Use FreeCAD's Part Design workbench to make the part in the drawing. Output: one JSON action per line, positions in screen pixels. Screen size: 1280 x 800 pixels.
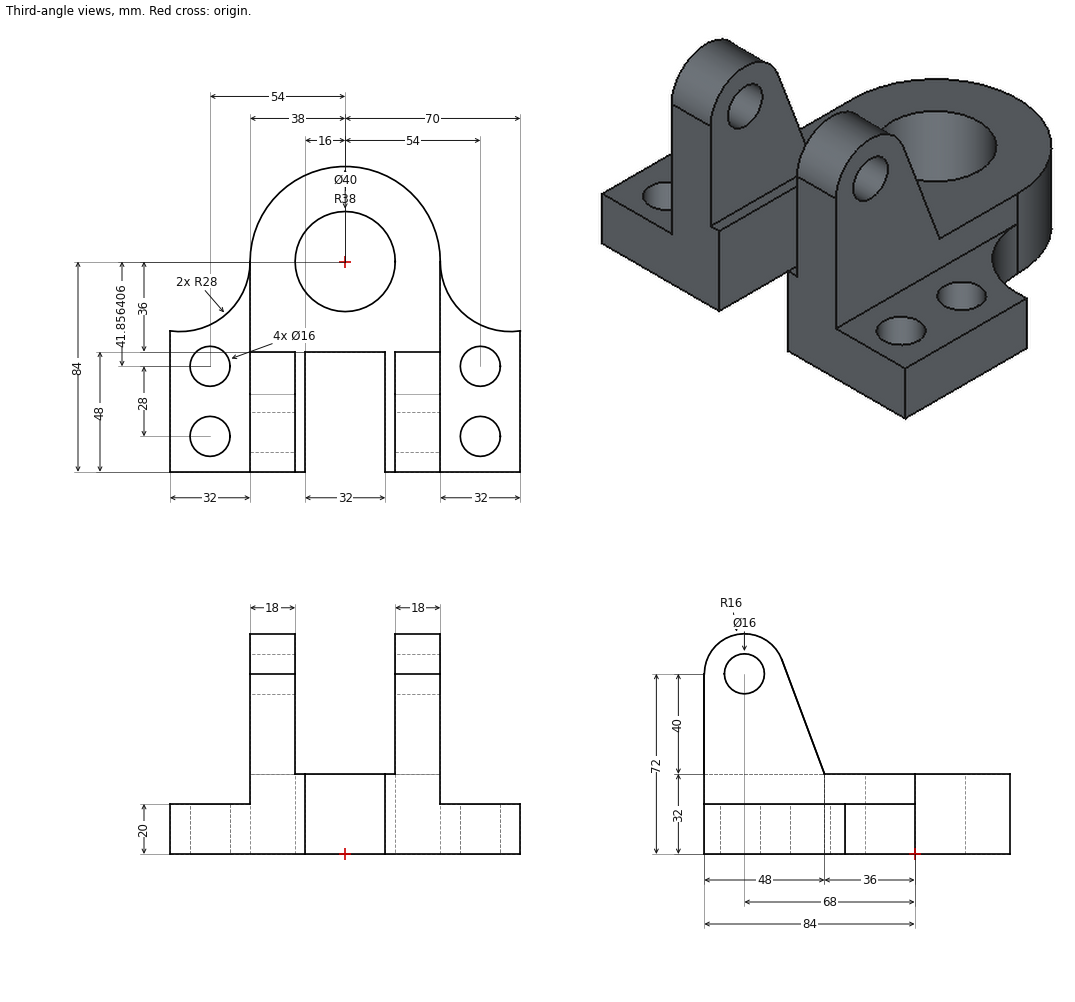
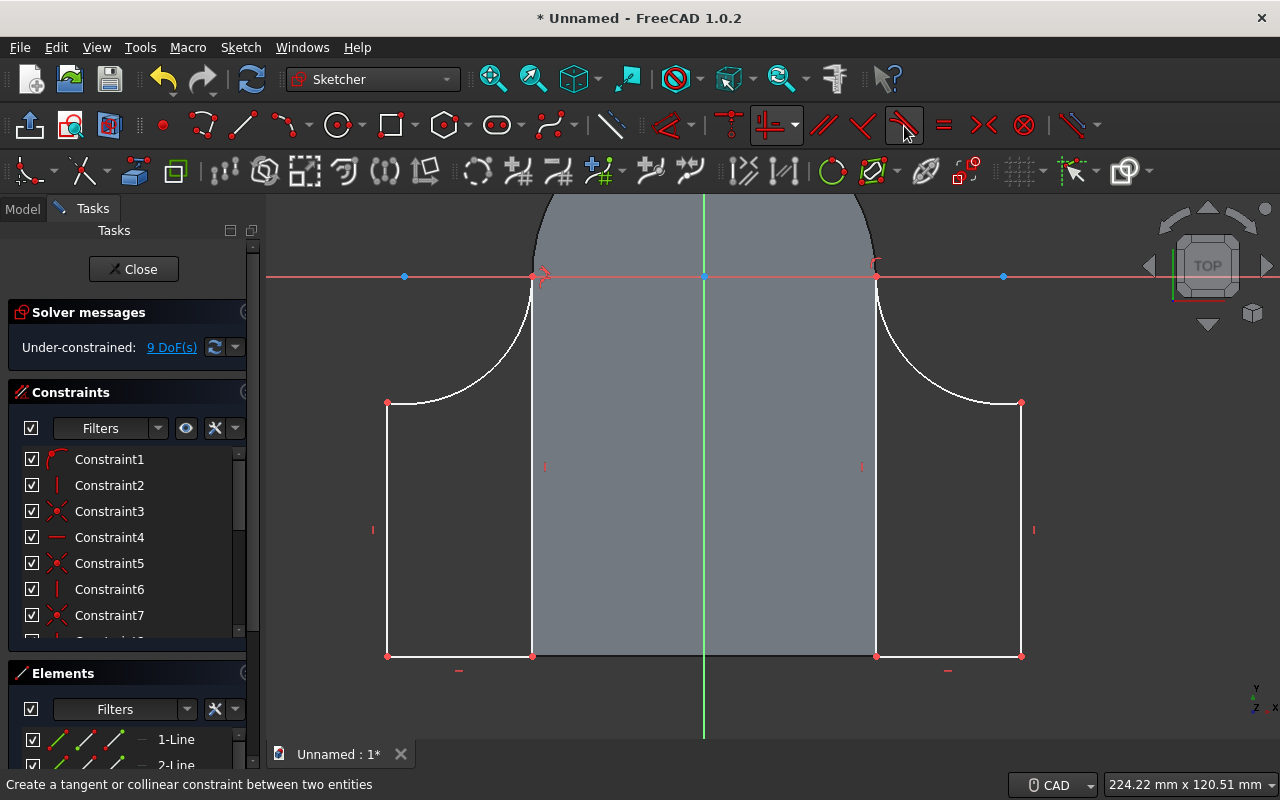
{"action": "left_click", "coordinate": [876, 543]}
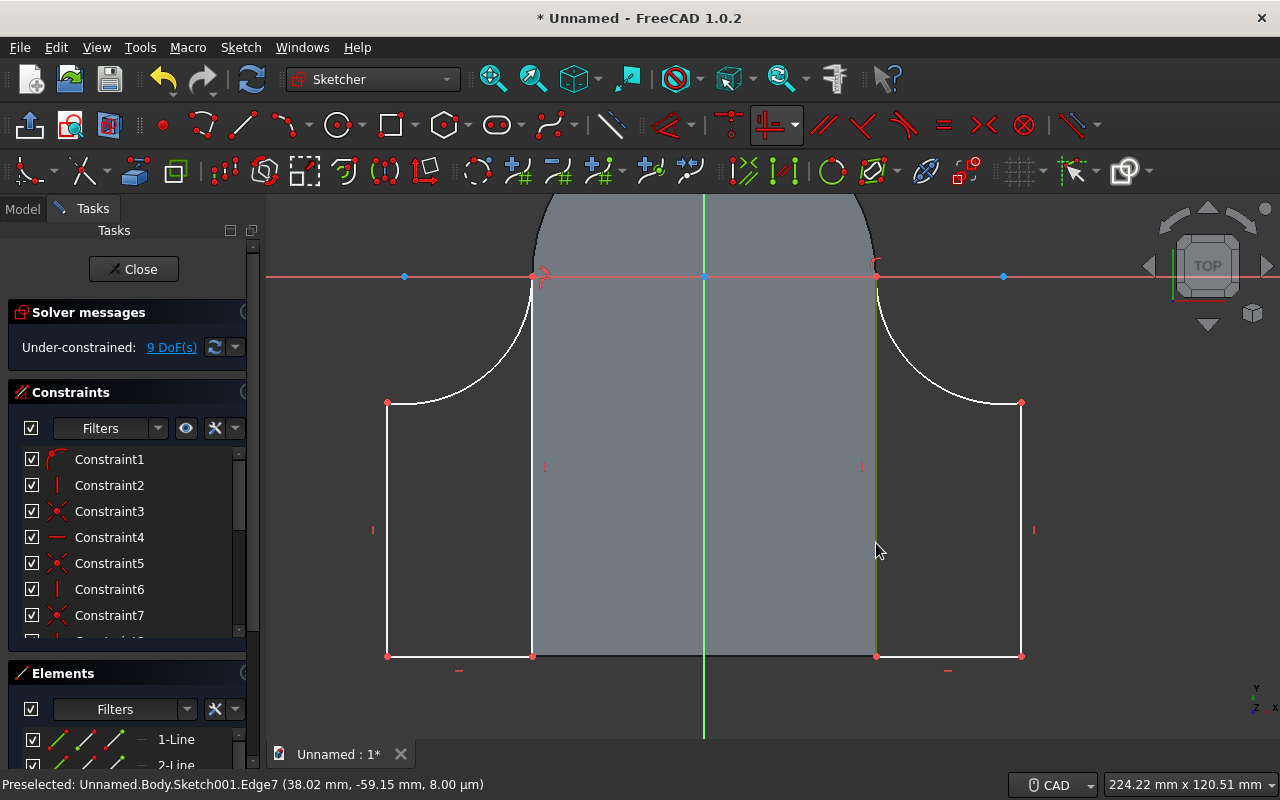
{"action": "left_click", "coordinate": [892, 339]}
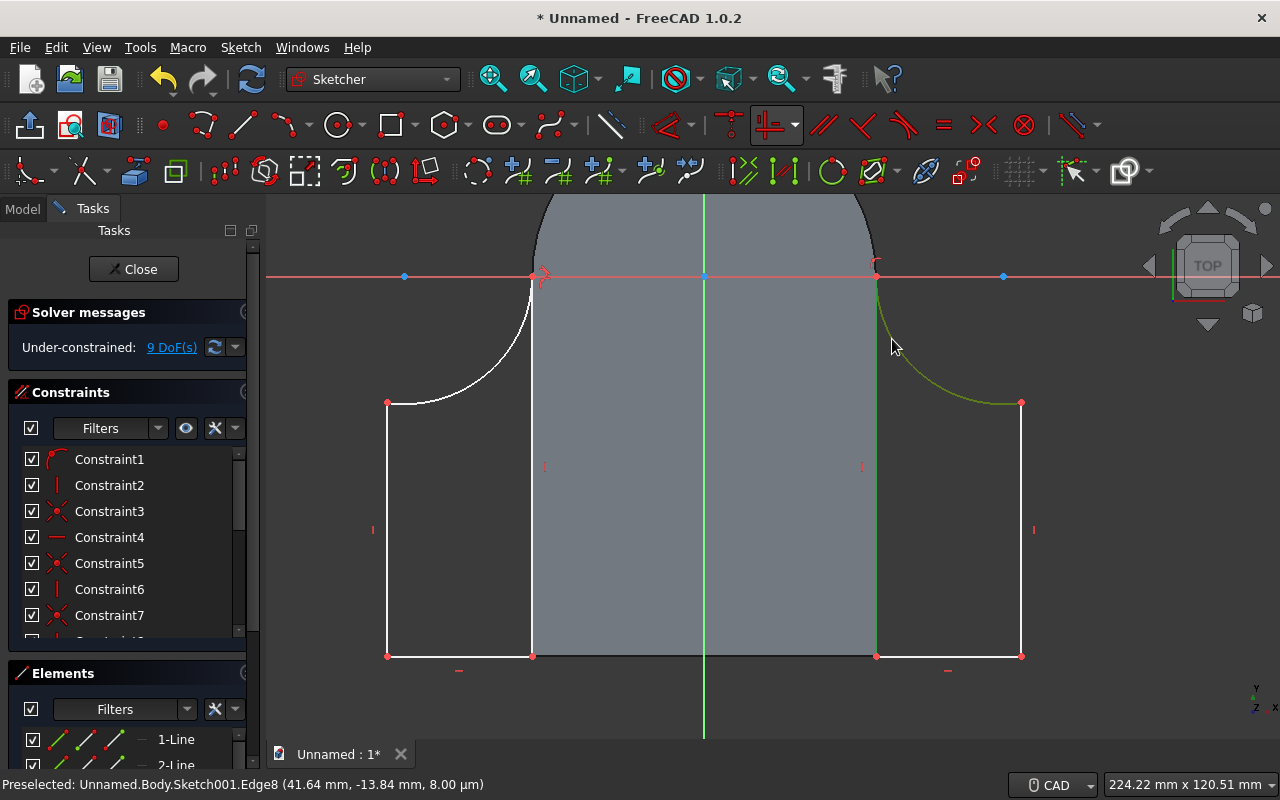
{"action": "left_click", "coordinate": [904, 126]}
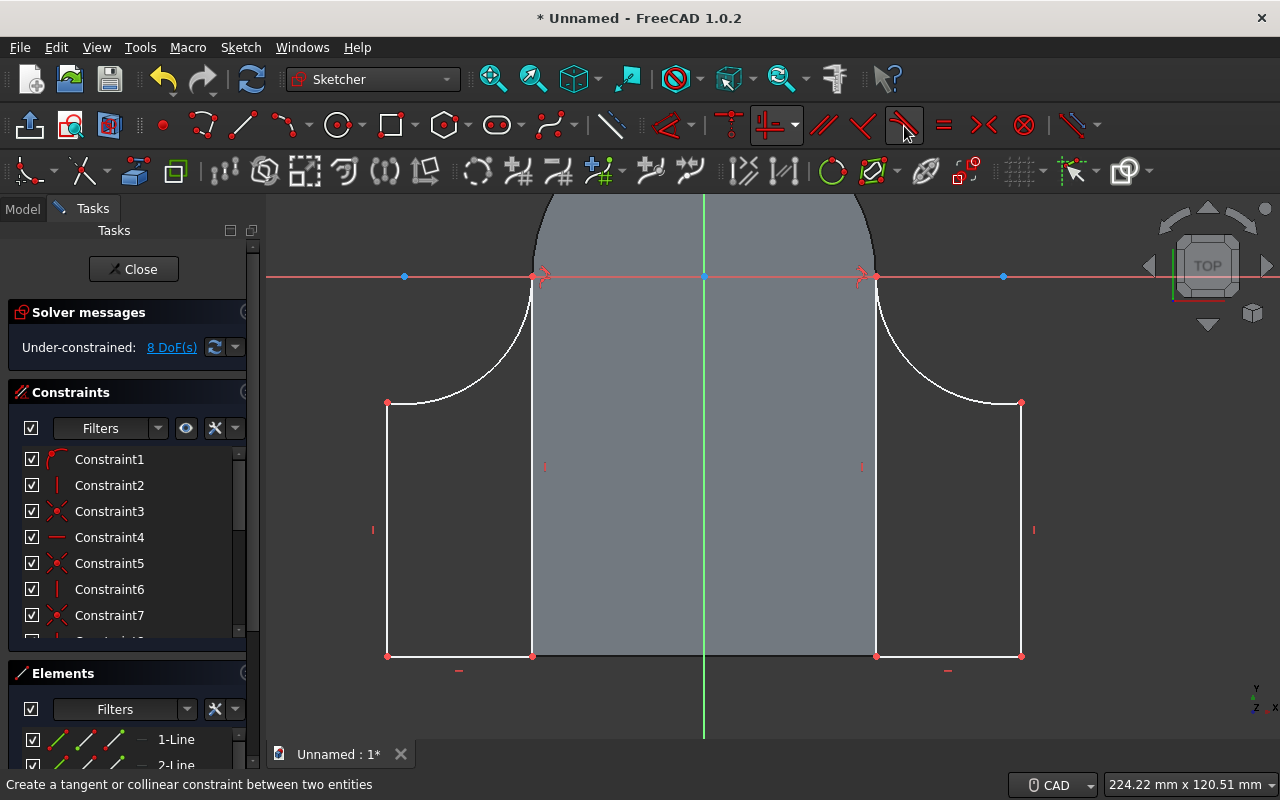
{"action": "left_click", "coordinate": [451, 395]}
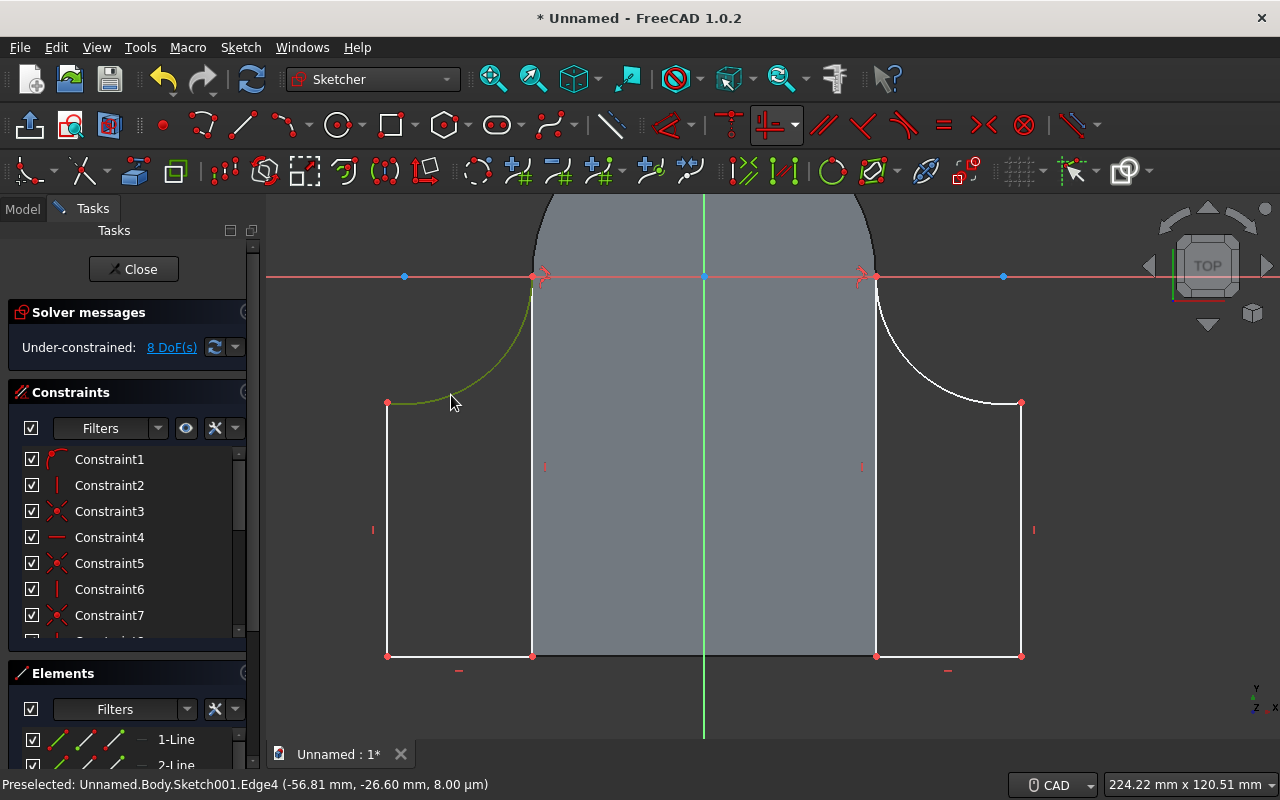
{"action": "left_click", "coordinate": [892, 339]}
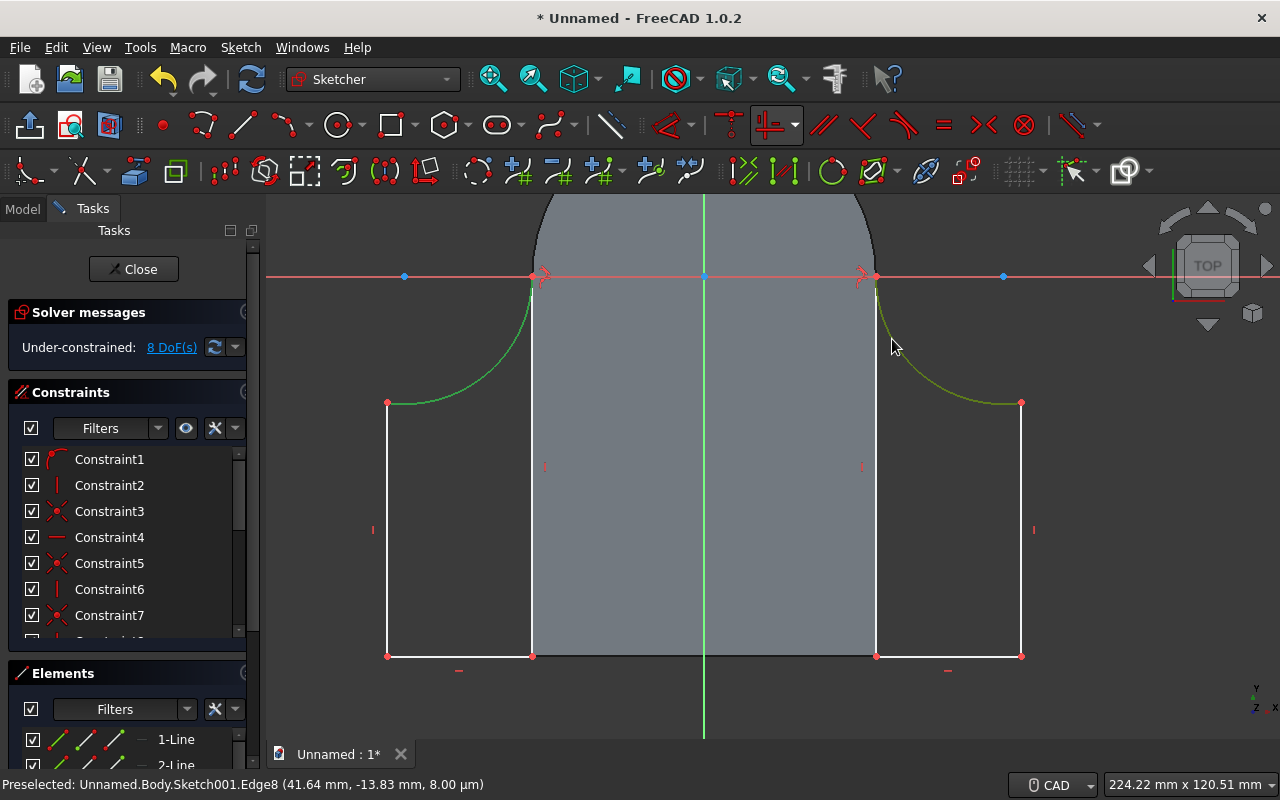
{"action": "left_click", "coordinate": [944, 126]}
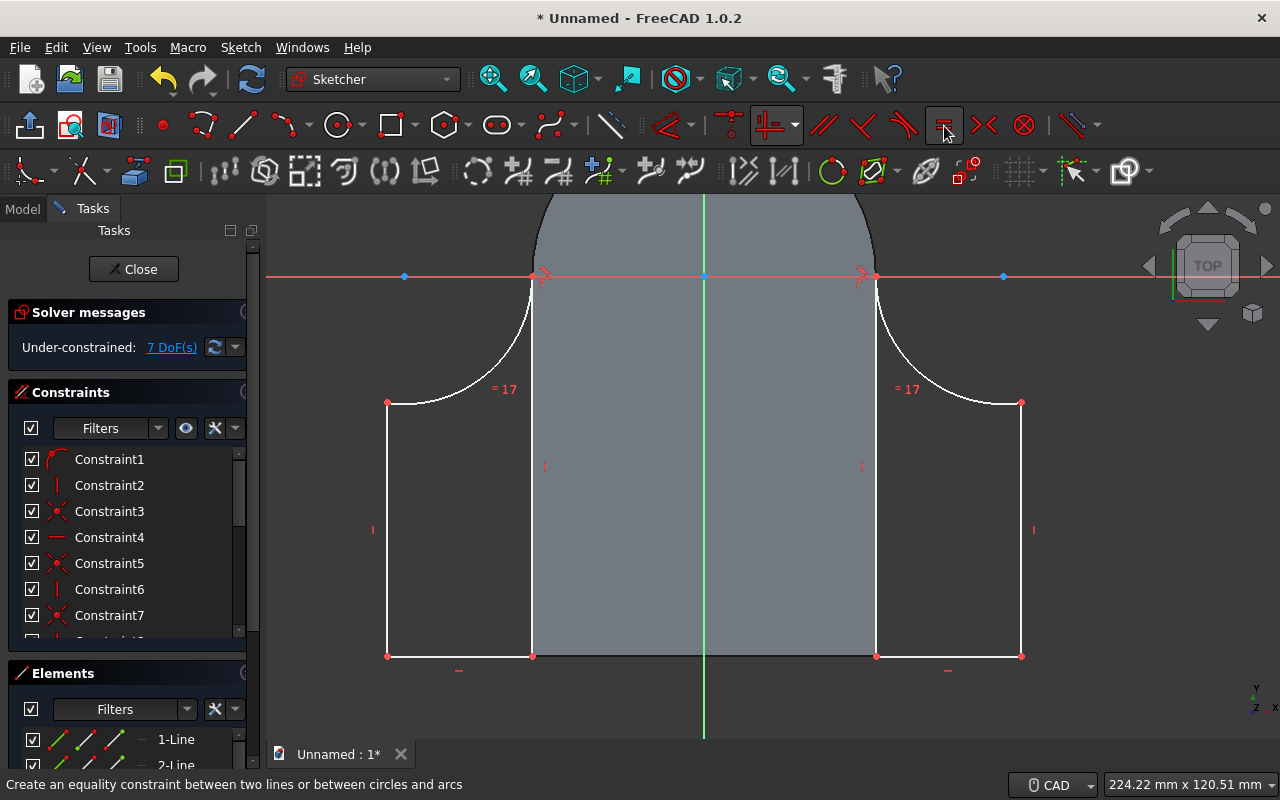
{"action": "left_click", "coordinate": [666, 126]}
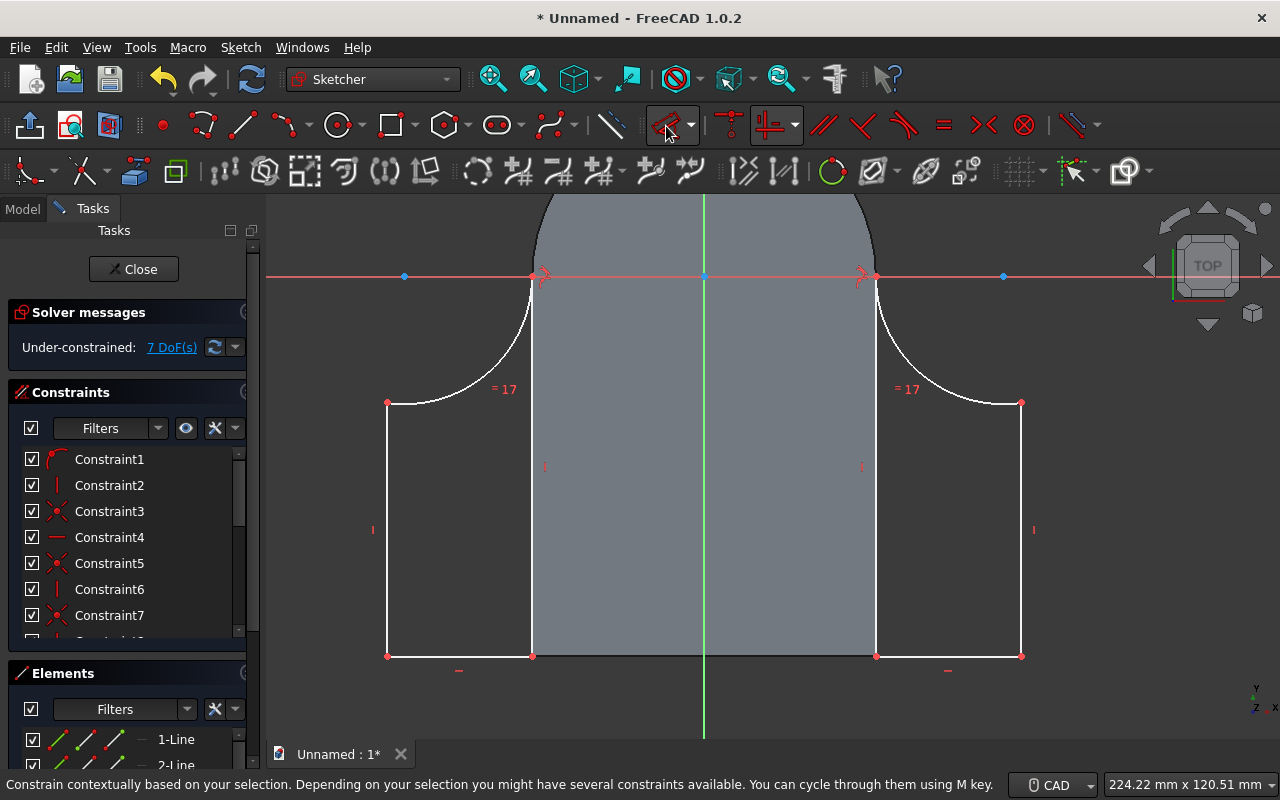
{"action": "left_click", "coordinate": [451, 395]}
{"action": "left_click", "coordinate": [463, 425]}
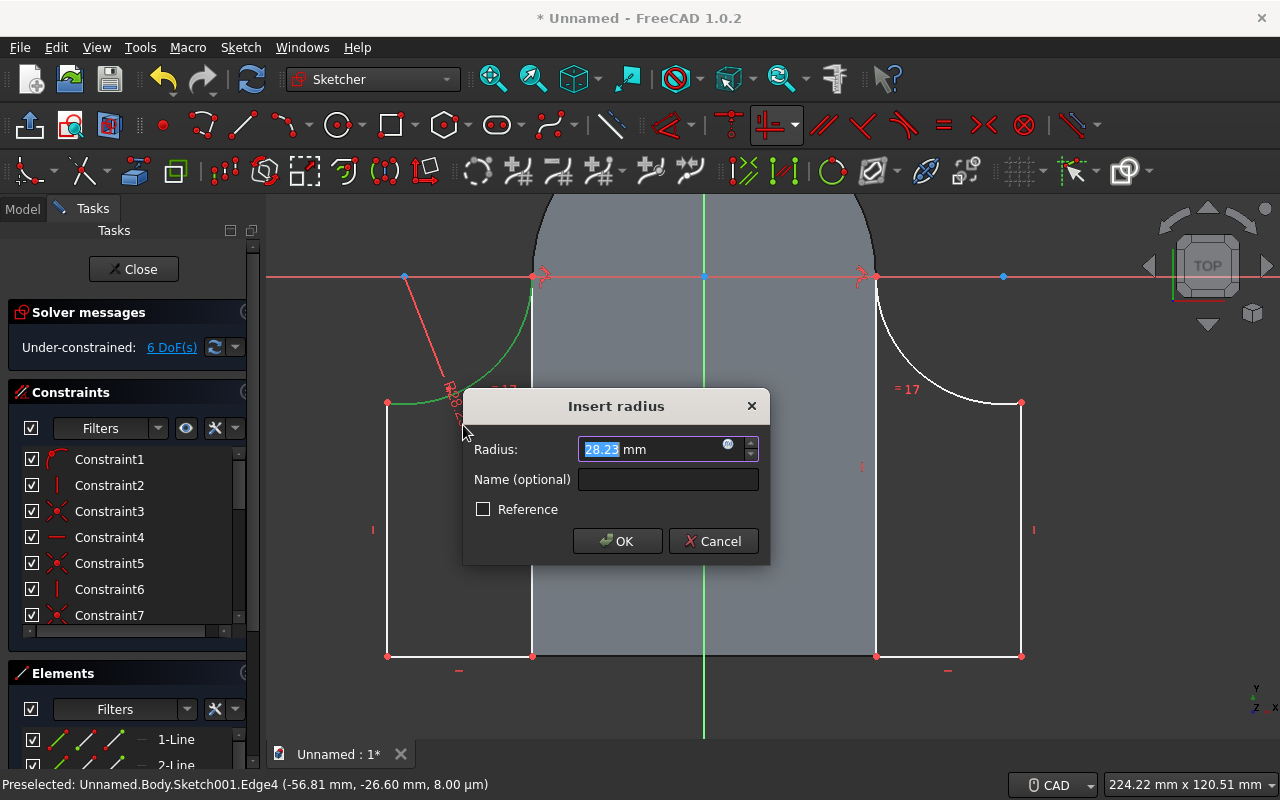
{"action": "type", "text": "28"}
{"action": "key", "text": "Return"}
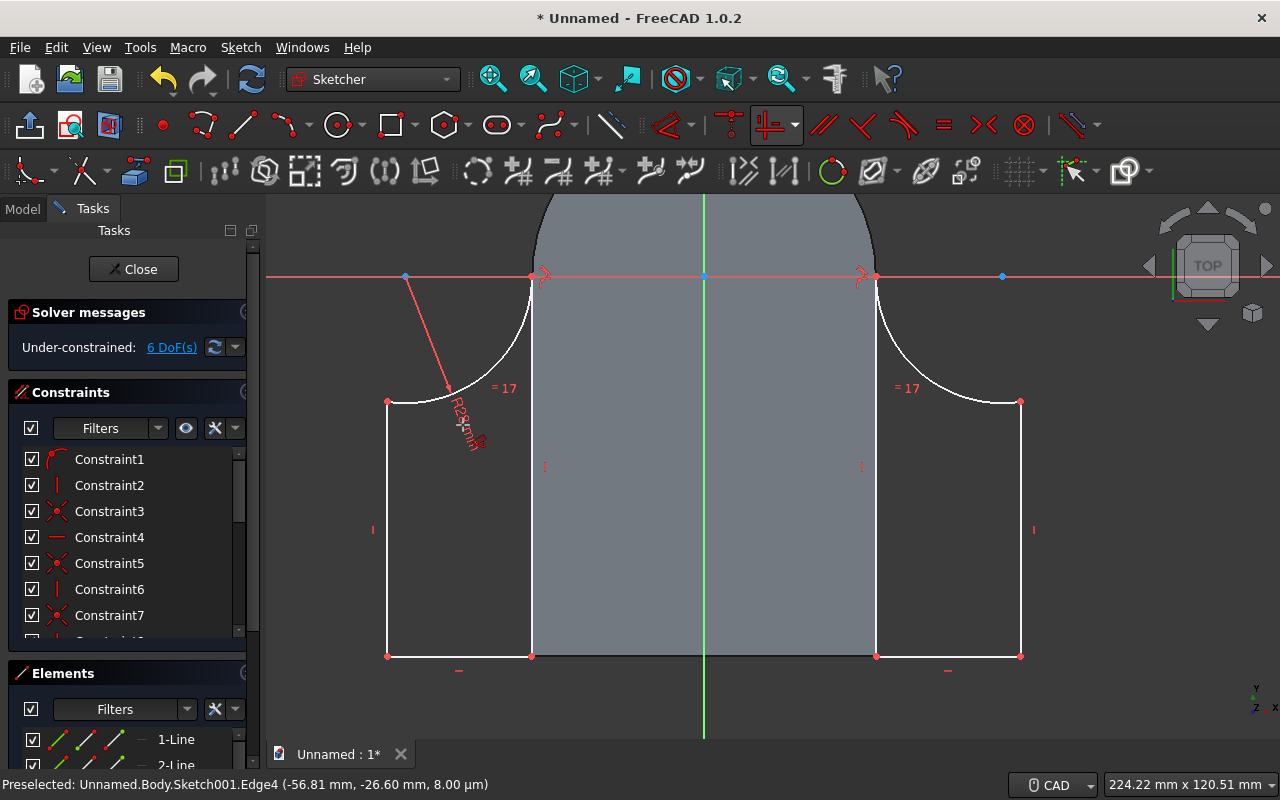
{"action": "left_click", "coordinate": [532, 391]}
{"action": "left_click", "coordinate": [498, 467]}